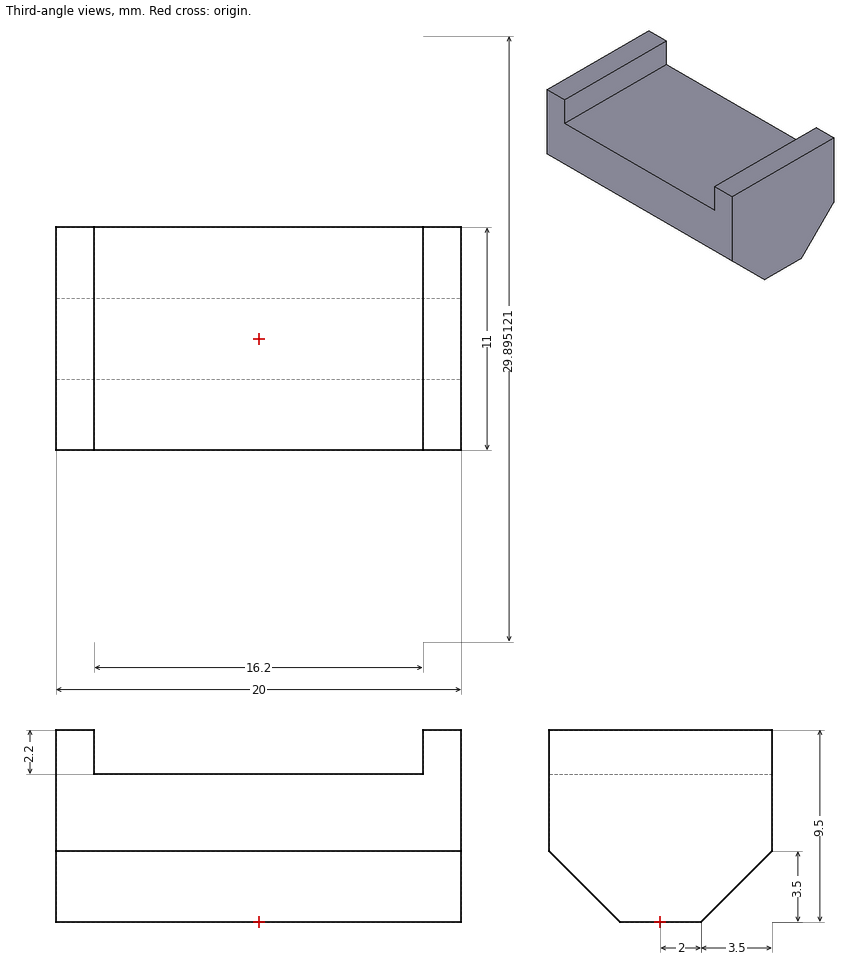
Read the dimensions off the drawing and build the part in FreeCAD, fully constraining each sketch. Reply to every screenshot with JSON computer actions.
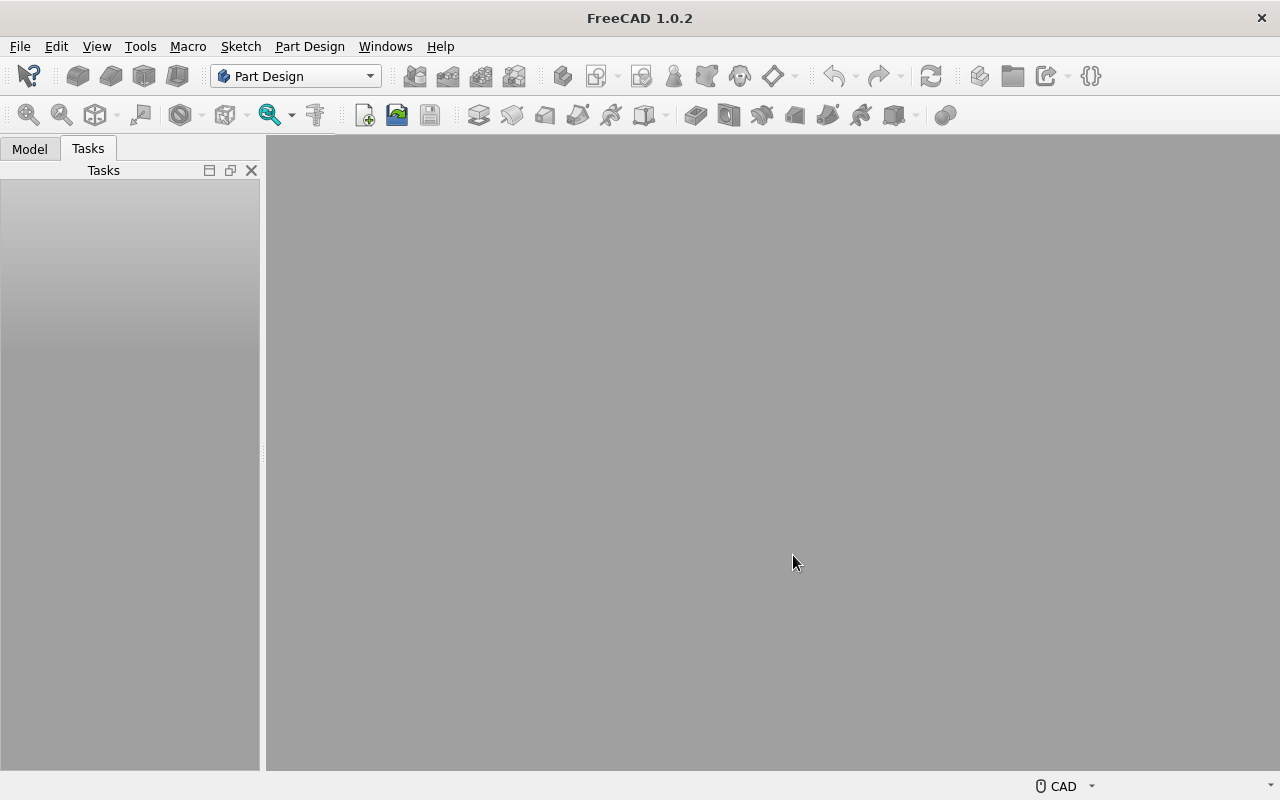
{"action": "left_click", "coordinate": [364, 116]}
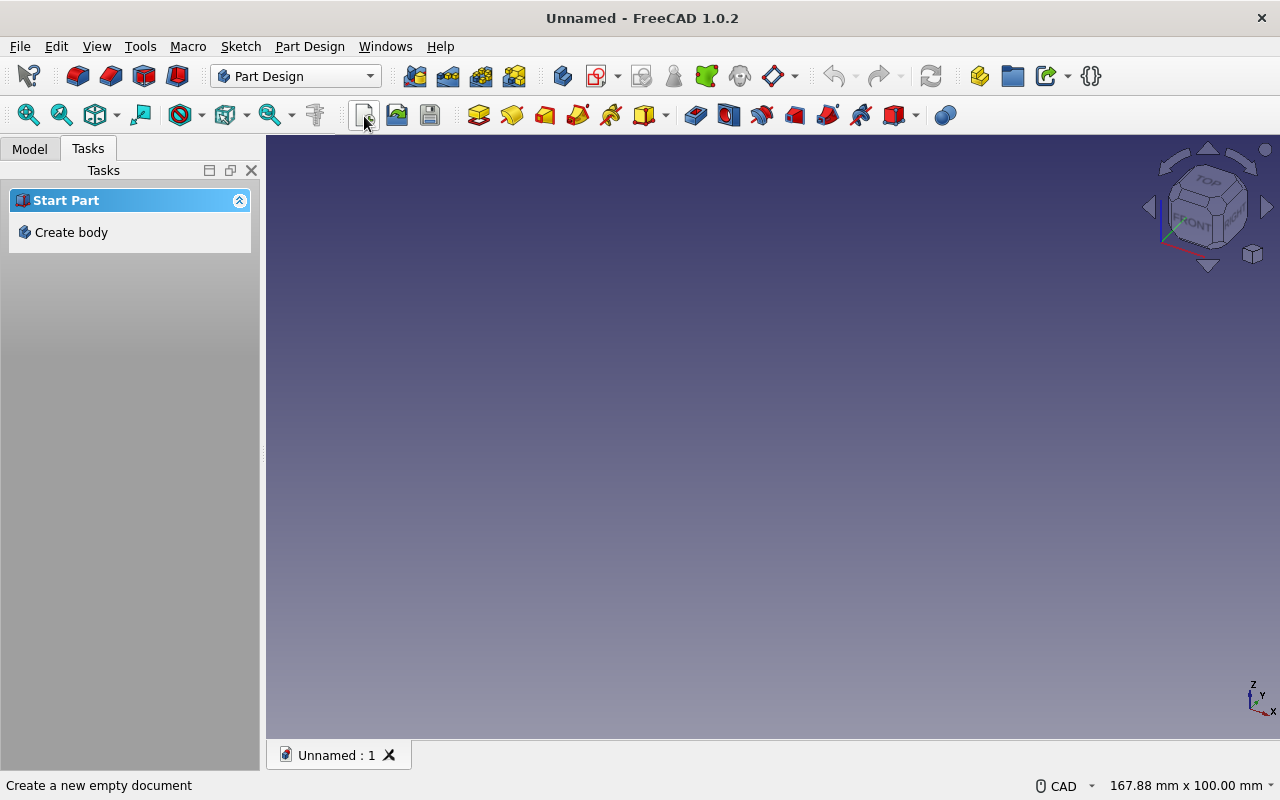
{"action": "left_click", "coordinate": [596, 76]}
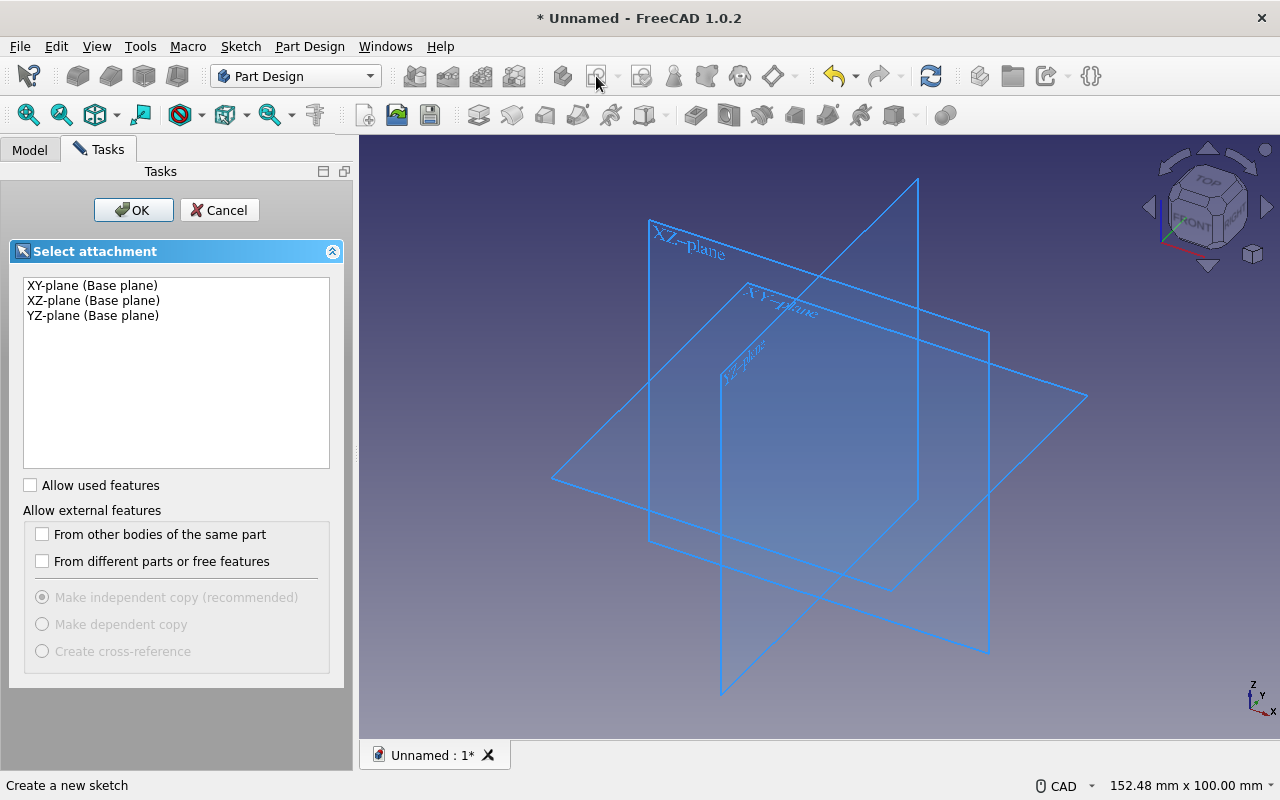
{"action": "left_click", "coordinate": [84, 286]}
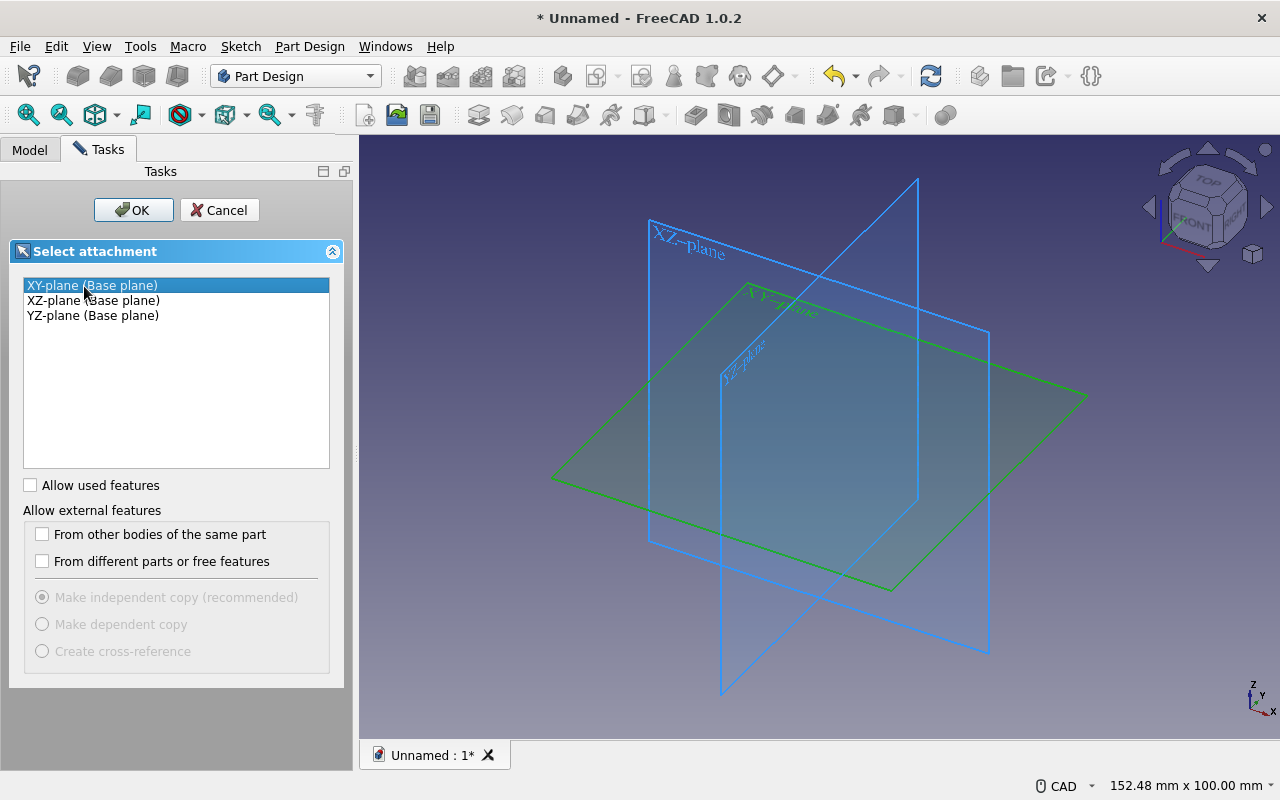
{"action": "left_click", "coordinate": [134, 210]}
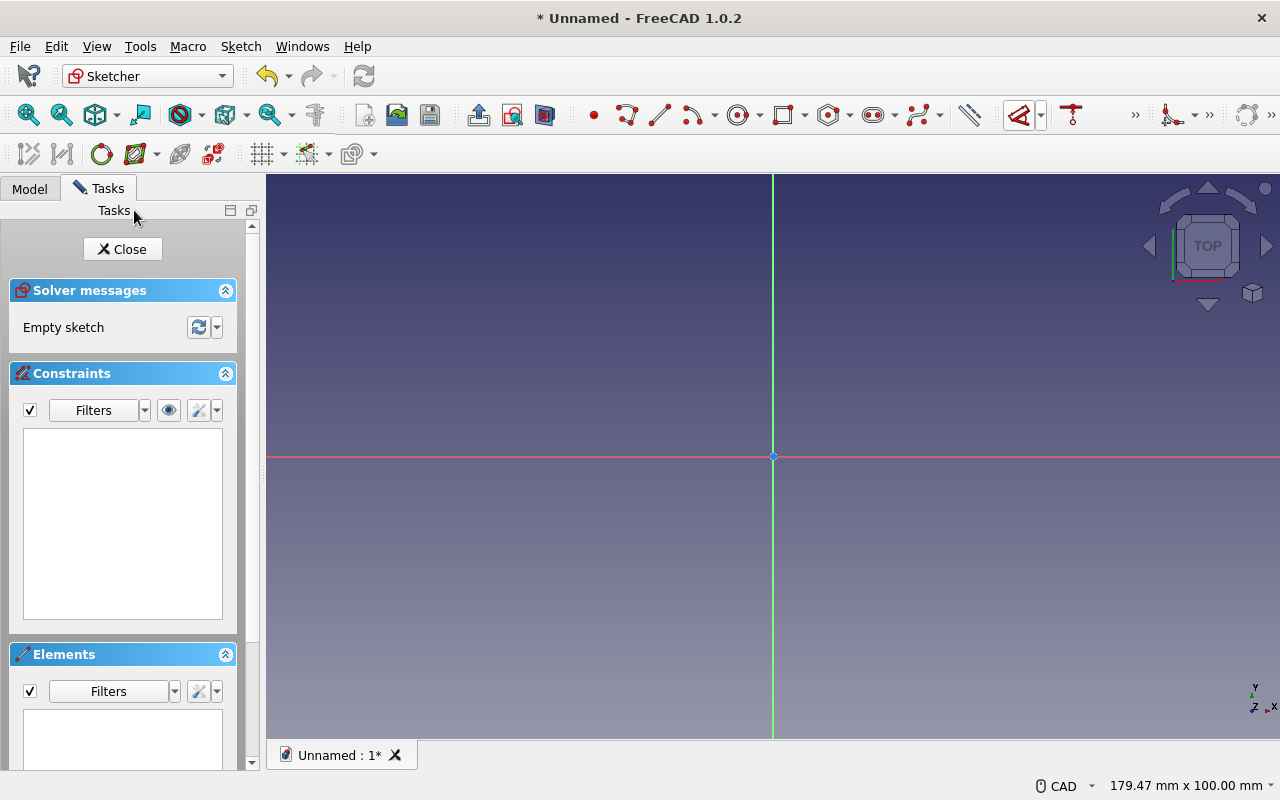
{"action": "scroll", "coordinate": [790, 456], "scroll_direction": "up", "scroll_amount": 8}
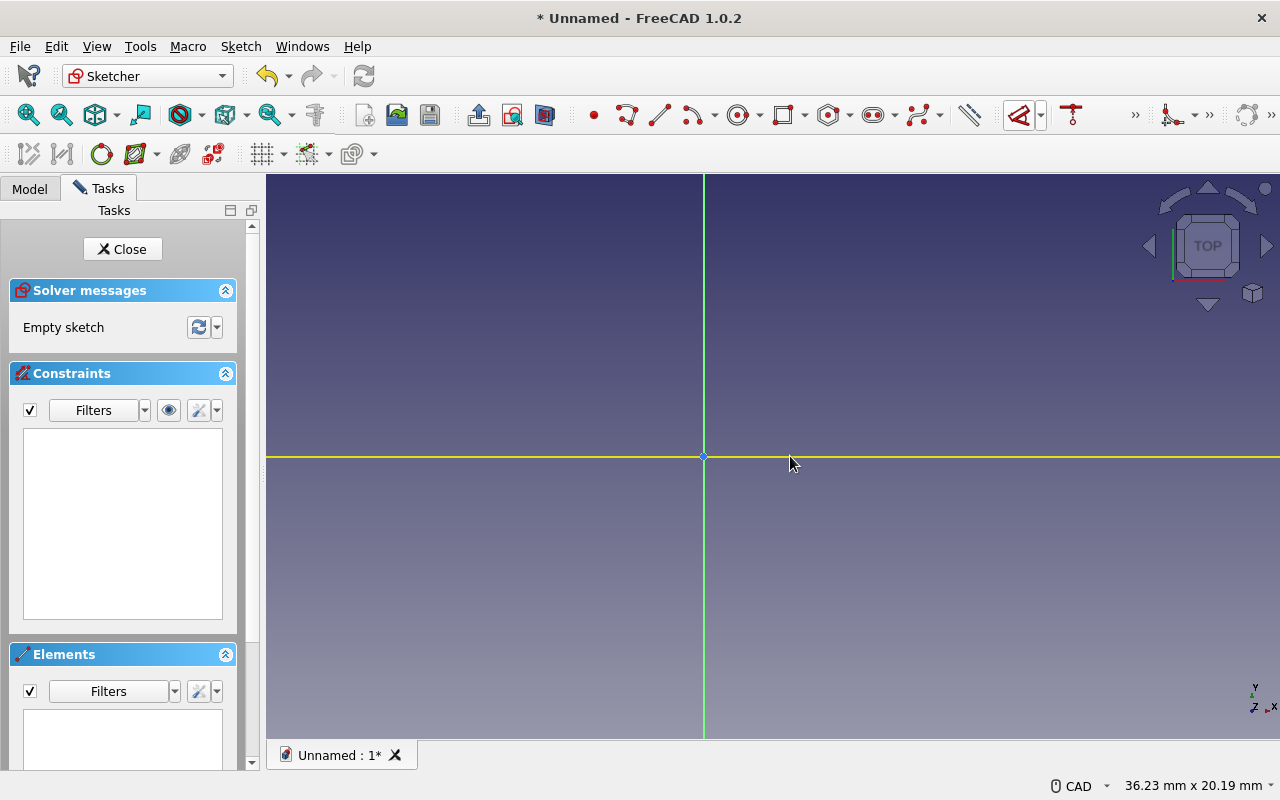
{"action": "key", "text": "g v"}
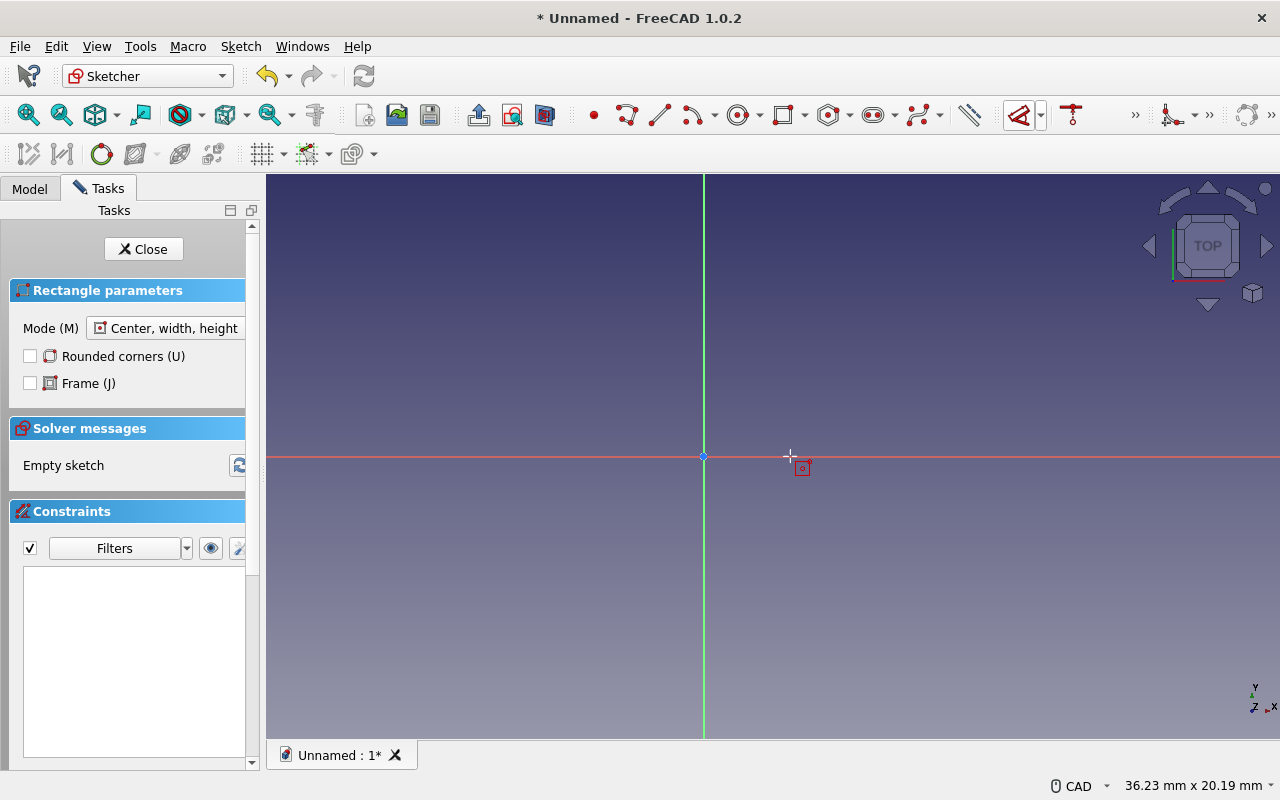
{"action": "left_click", "coordinate": [704, 456]}
{"action": "mouse_move", "coordinate": [984, 303]}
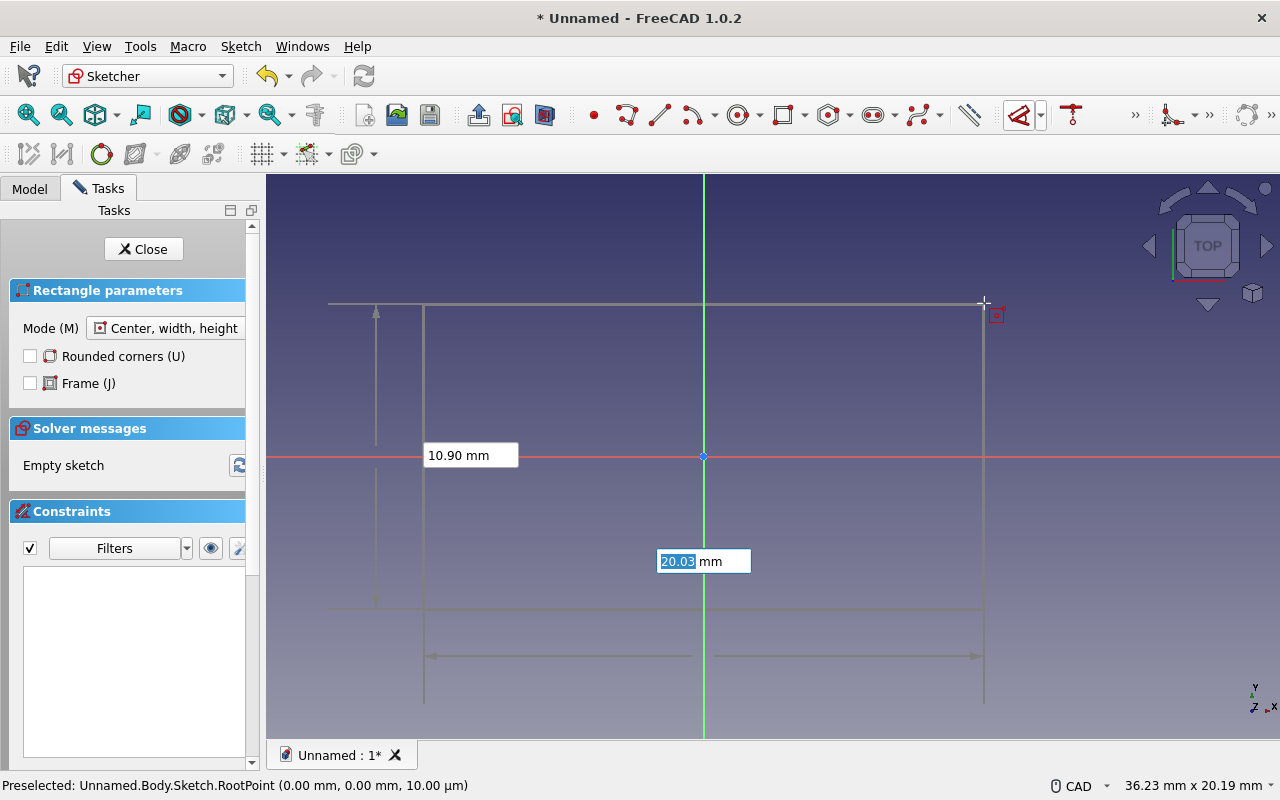
{"action": "type", "text": "20"}
{"action": "key", "text": "Tab"}
{"action": "type", "text": "11"}
{"action": "key", "text": "Return"}
{"action": "key", "text": "Escape"}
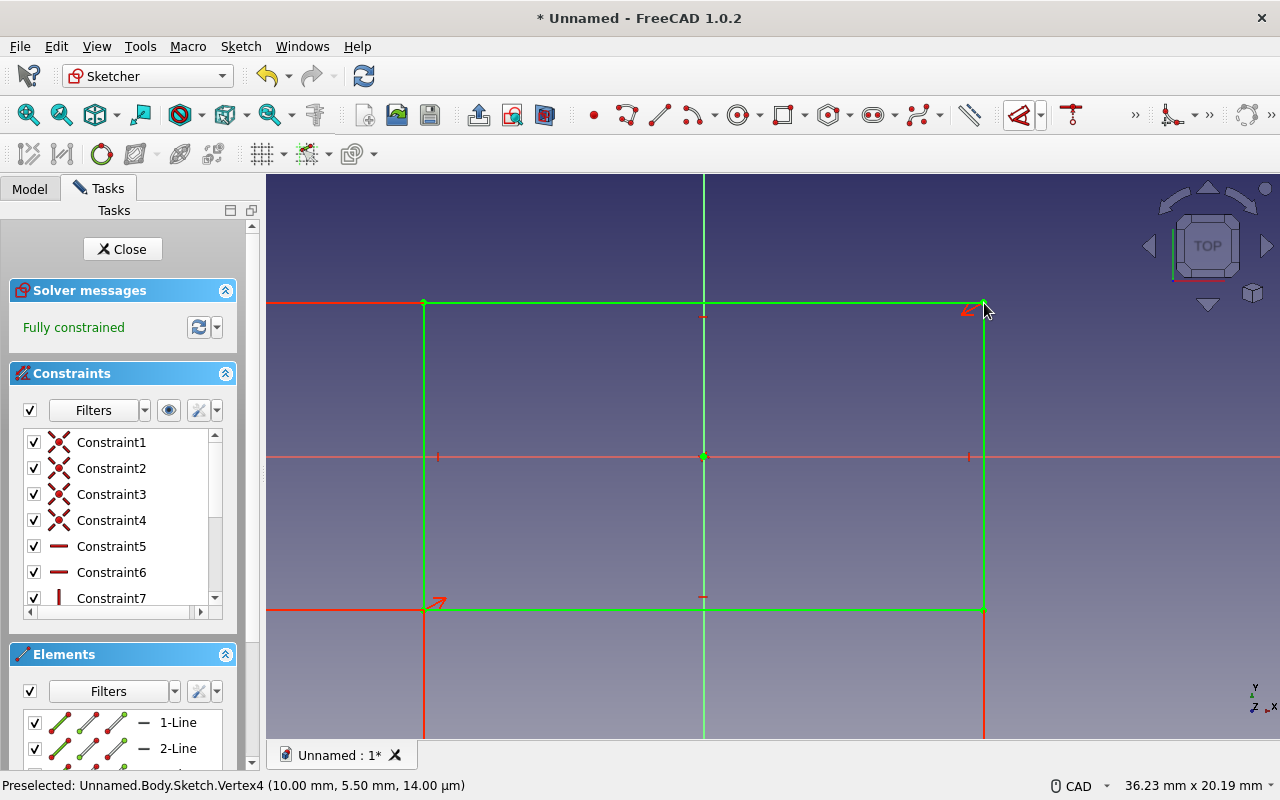
{"action": "left_click", "coordinate": [123, 249]}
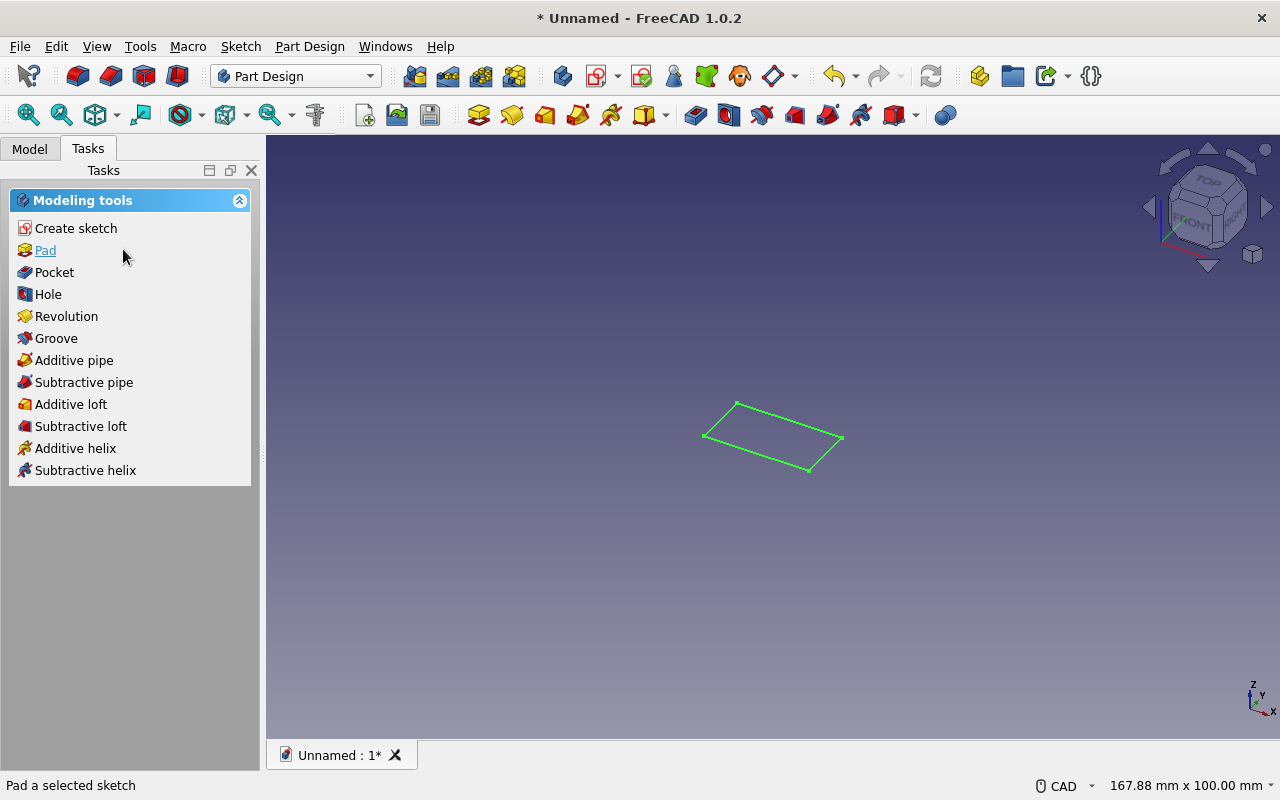
{"action": "left_click", "coordinate": [479, 116]}